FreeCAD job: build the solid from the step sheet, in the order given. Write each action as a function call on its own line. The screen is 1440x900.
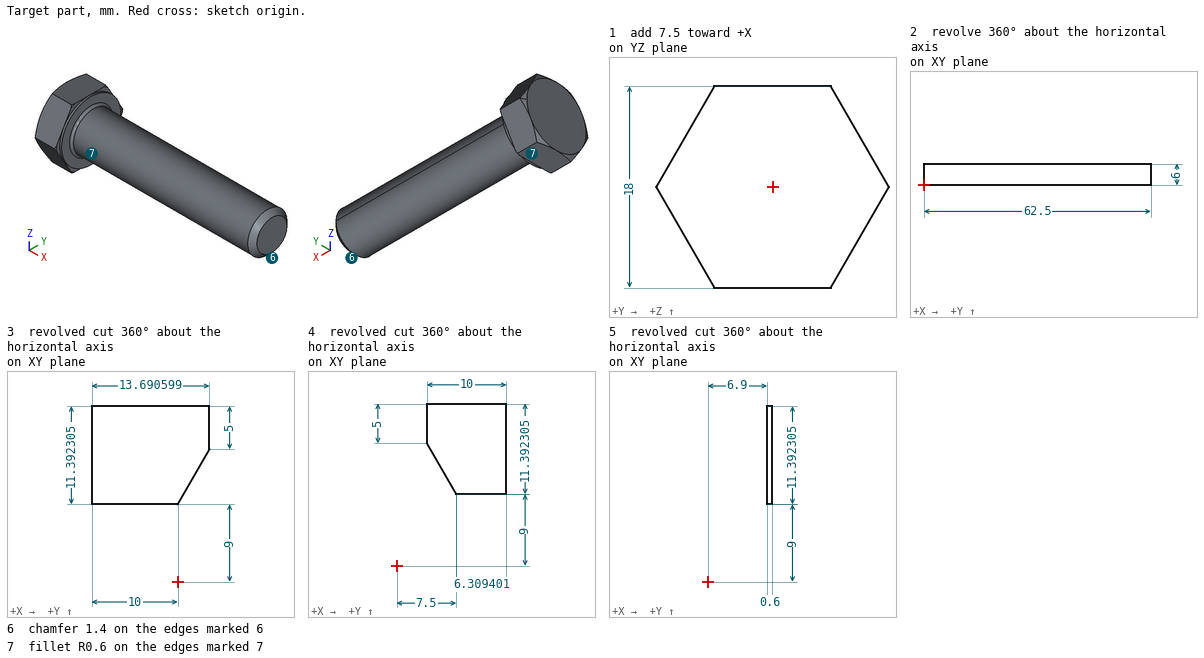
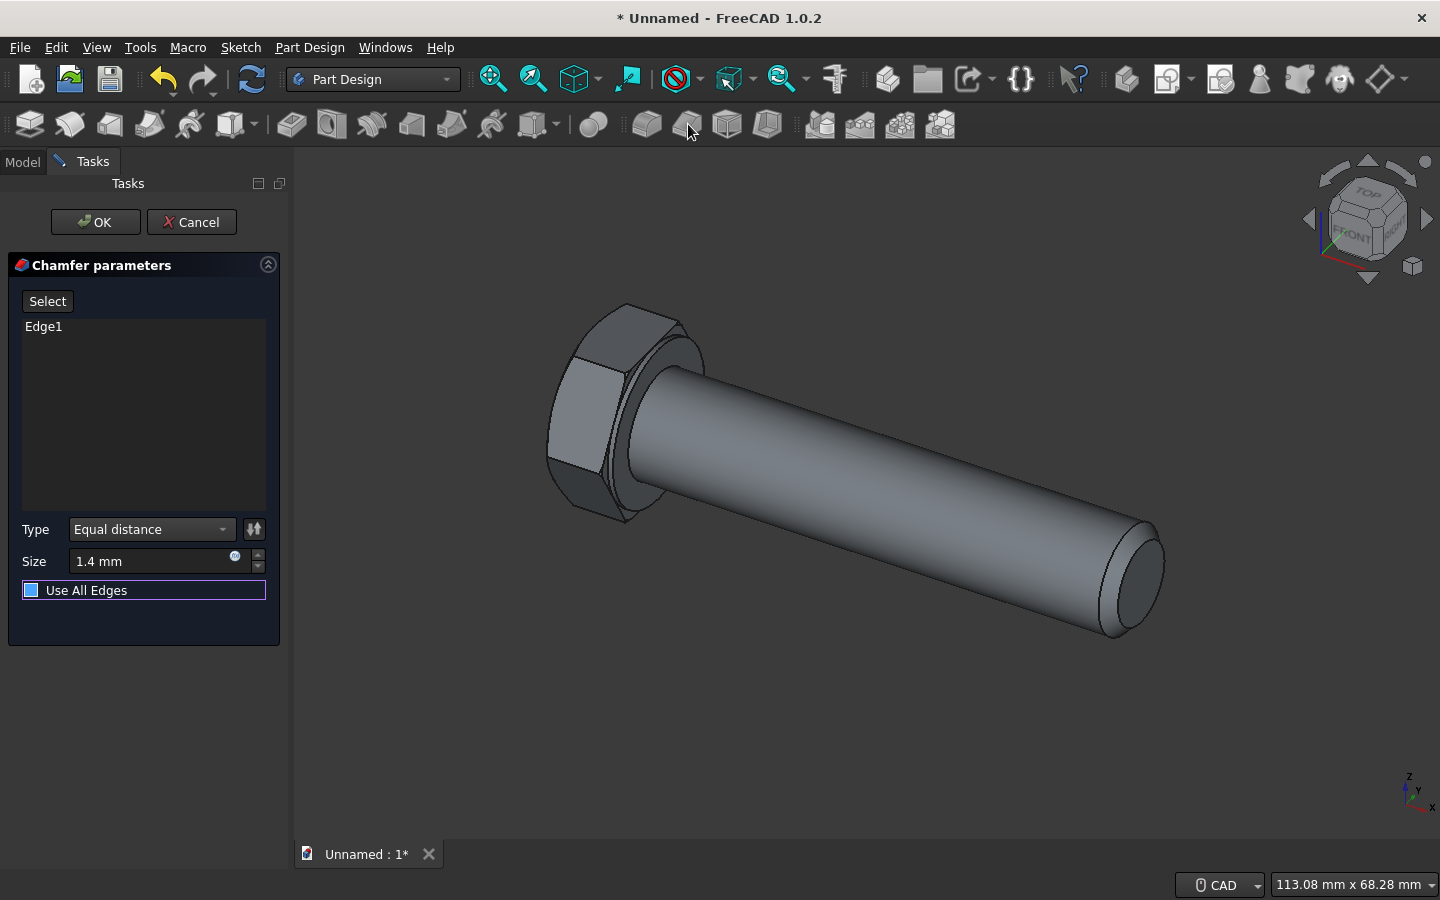
click(96, 222)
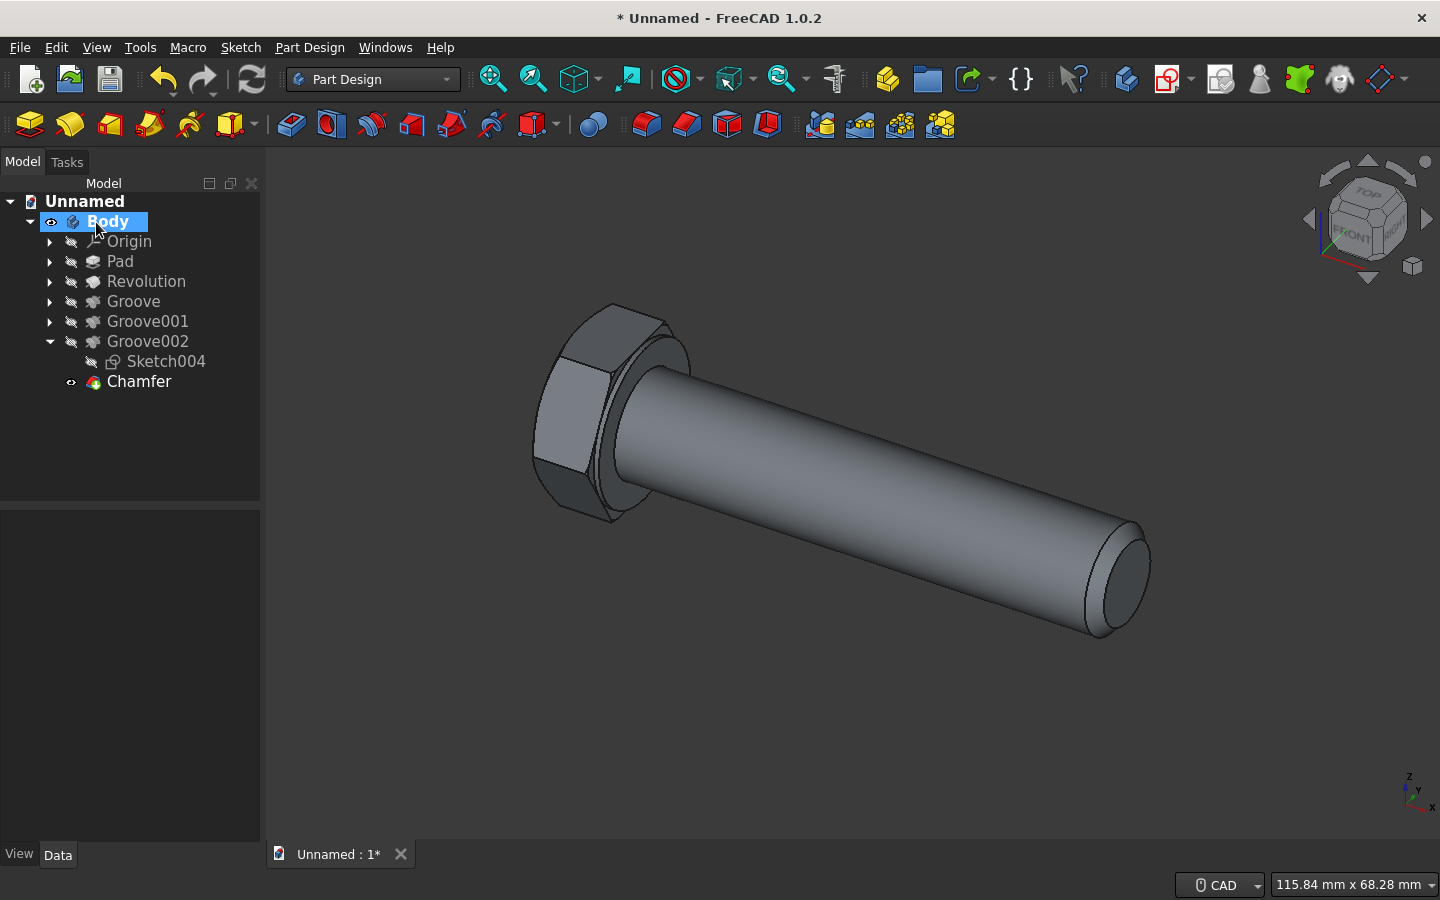
key(0)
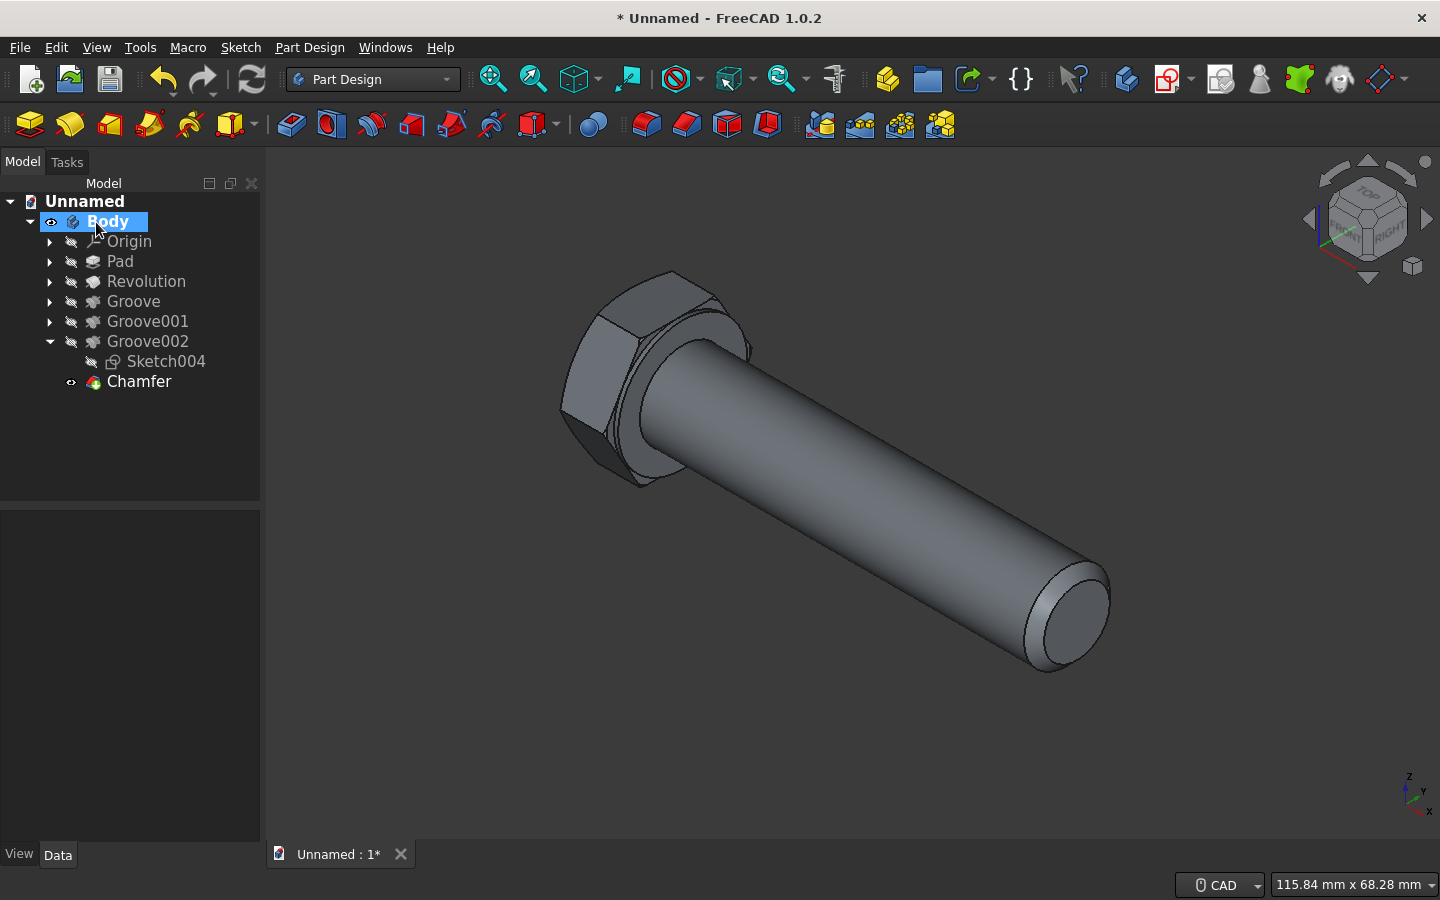
key(2)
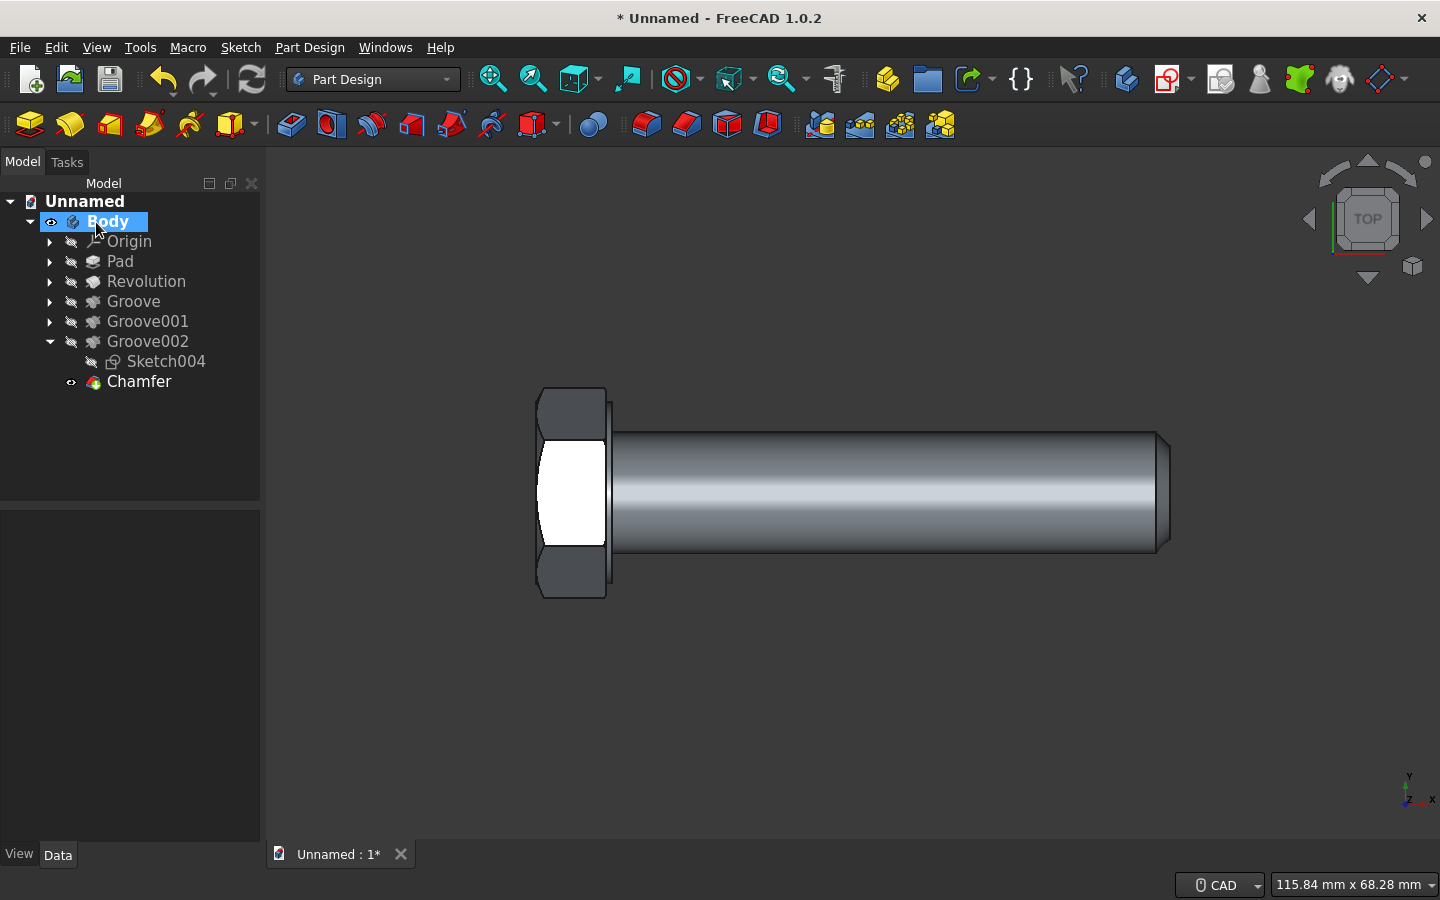
key(1)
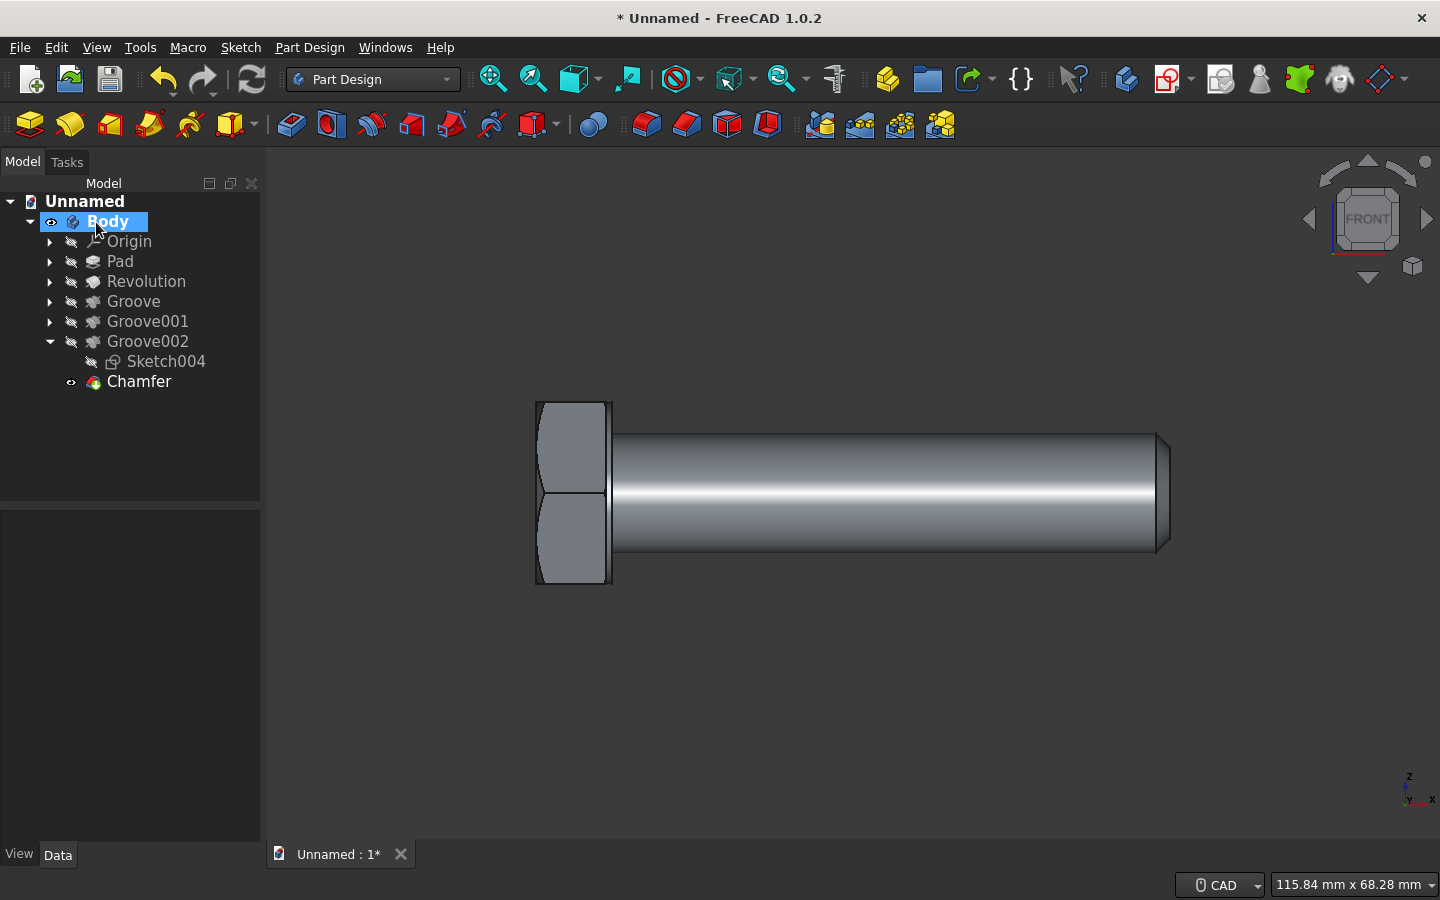
key(3)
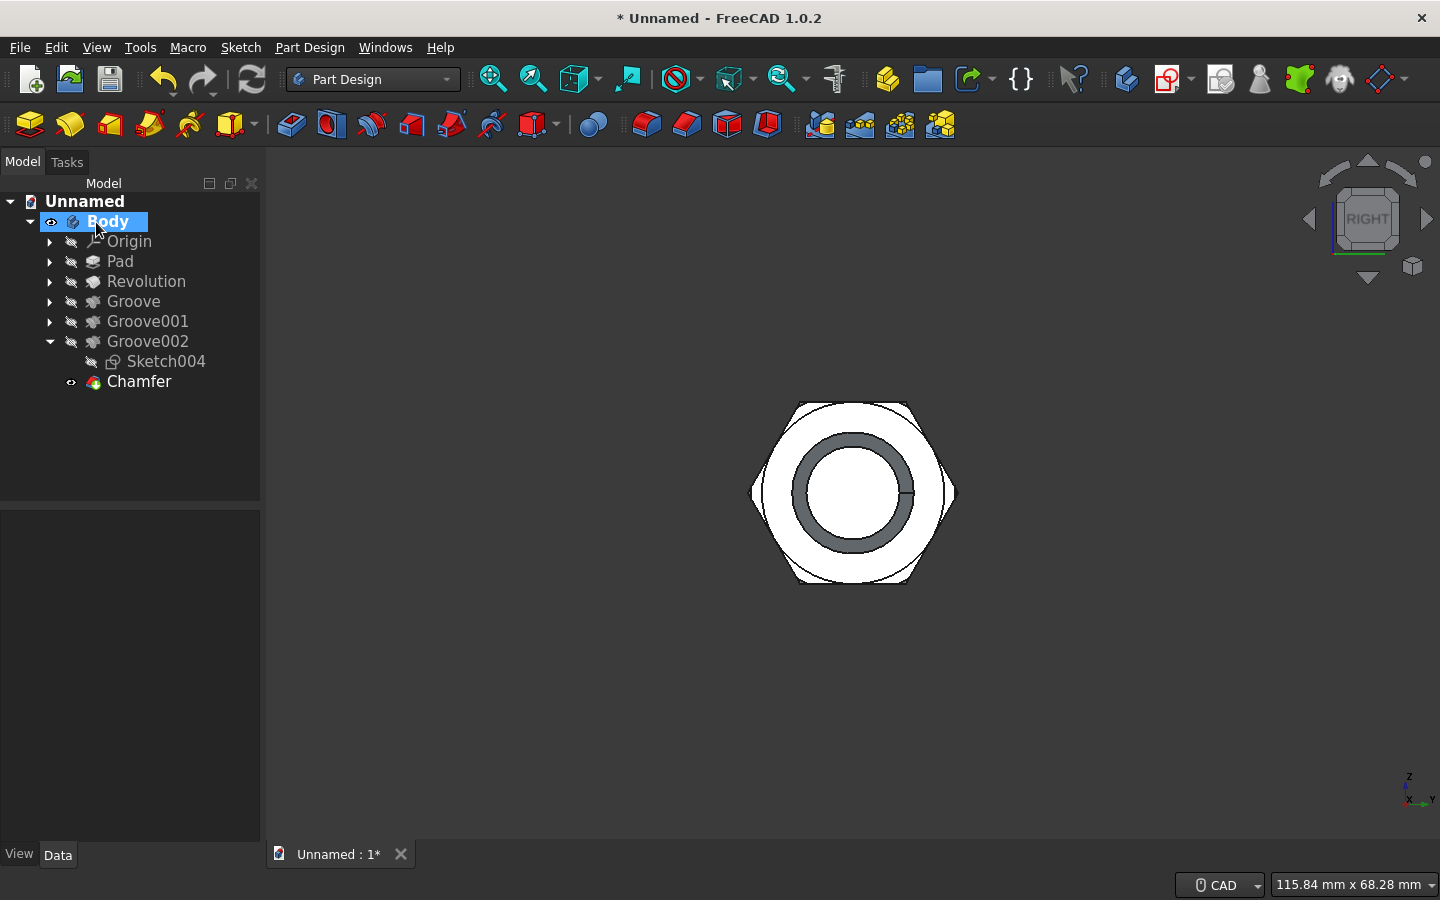
click(494, 80)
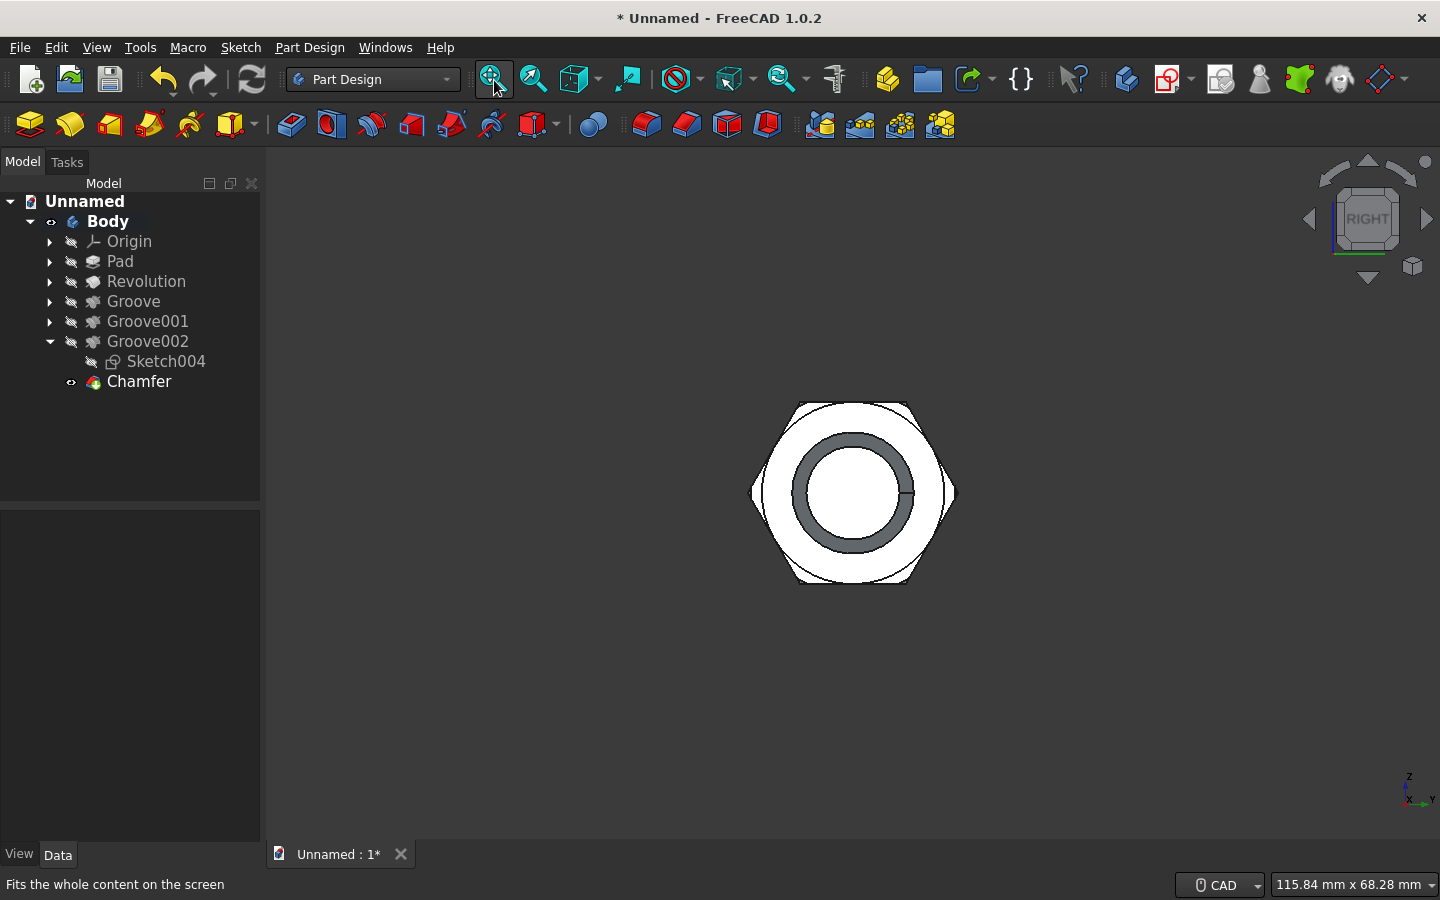
key(5)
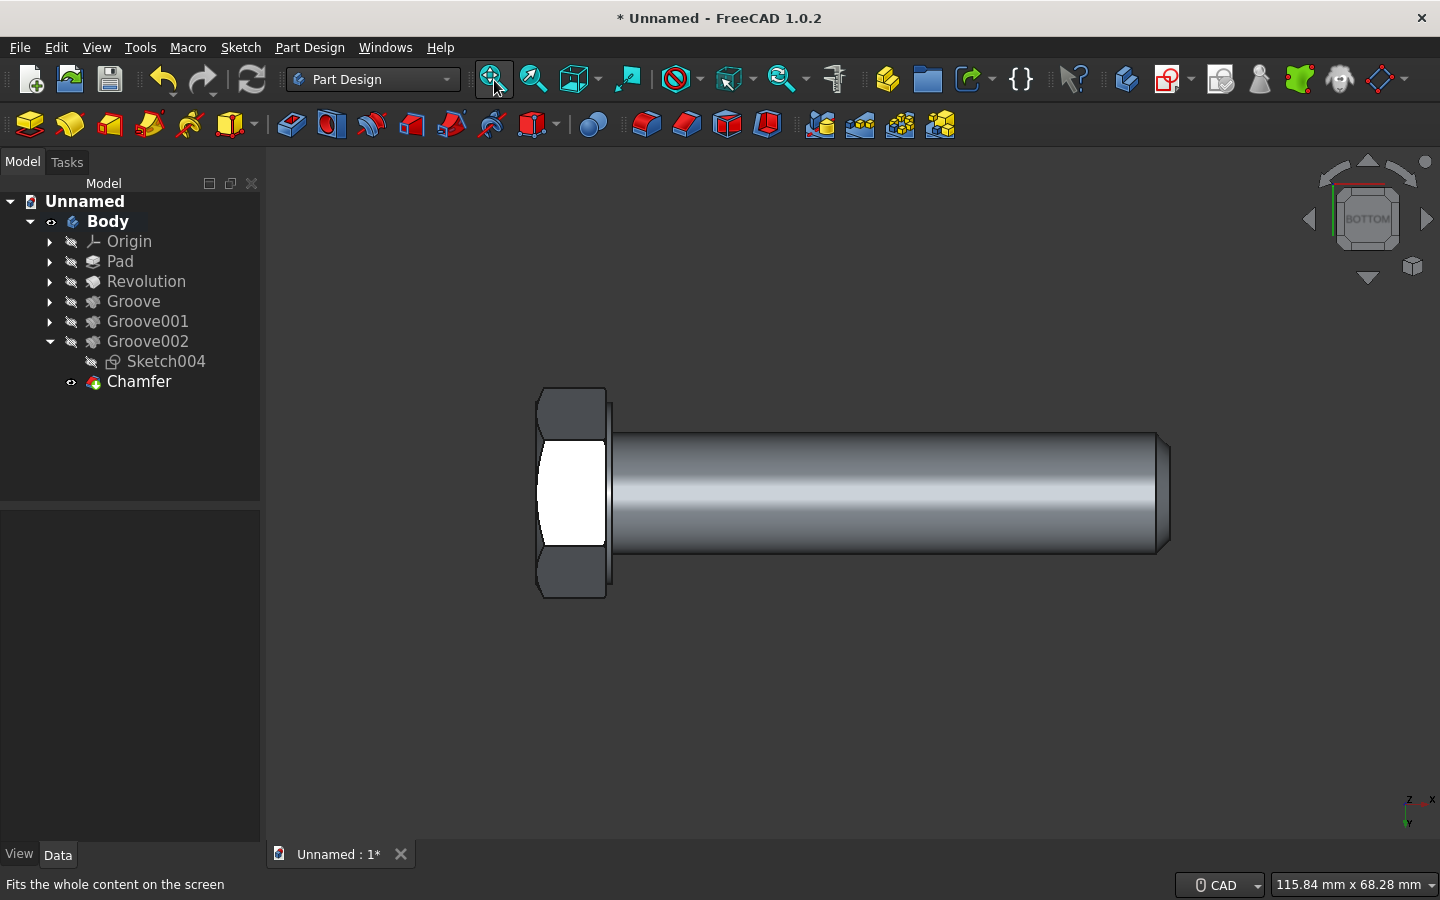
key(4)